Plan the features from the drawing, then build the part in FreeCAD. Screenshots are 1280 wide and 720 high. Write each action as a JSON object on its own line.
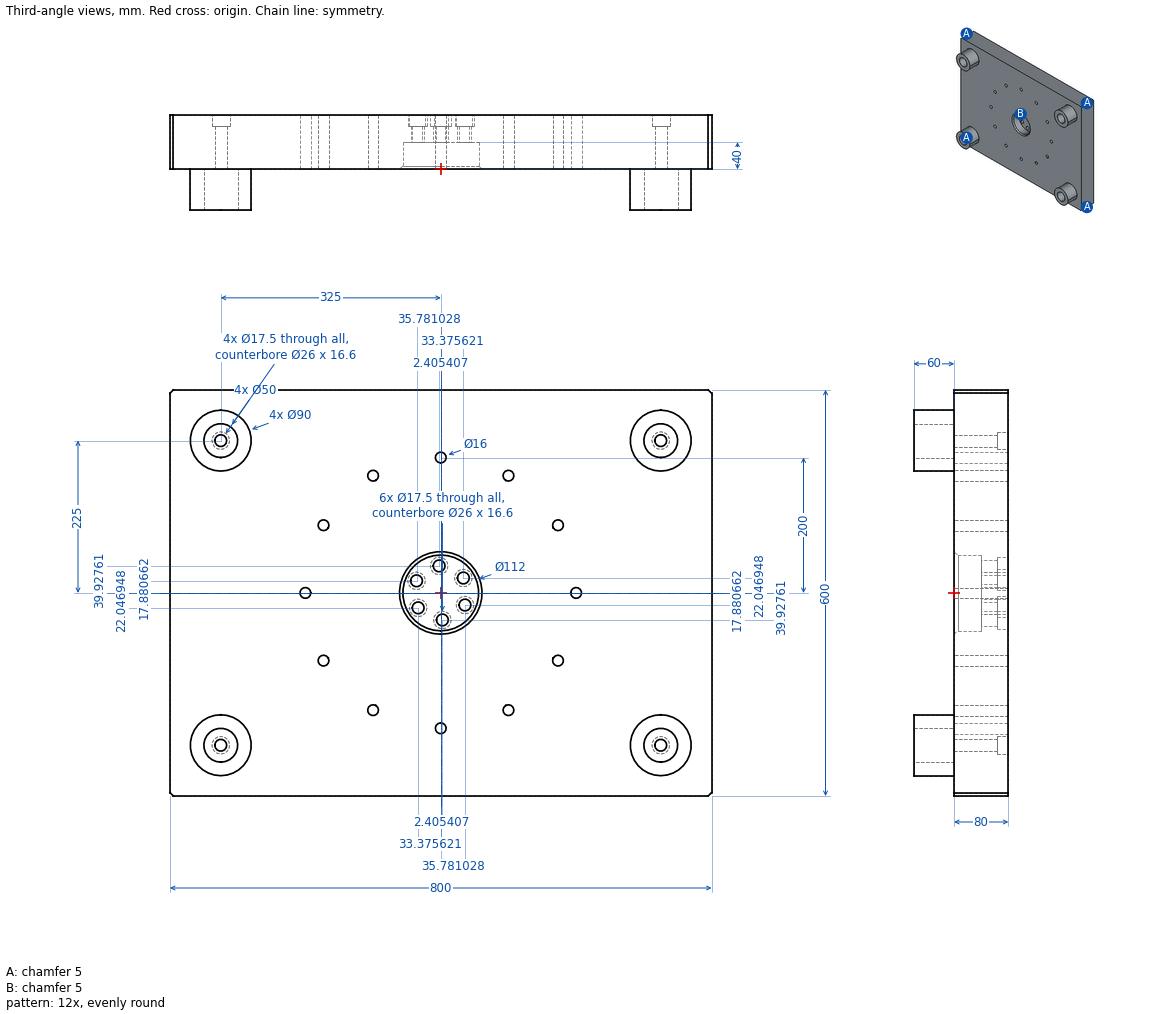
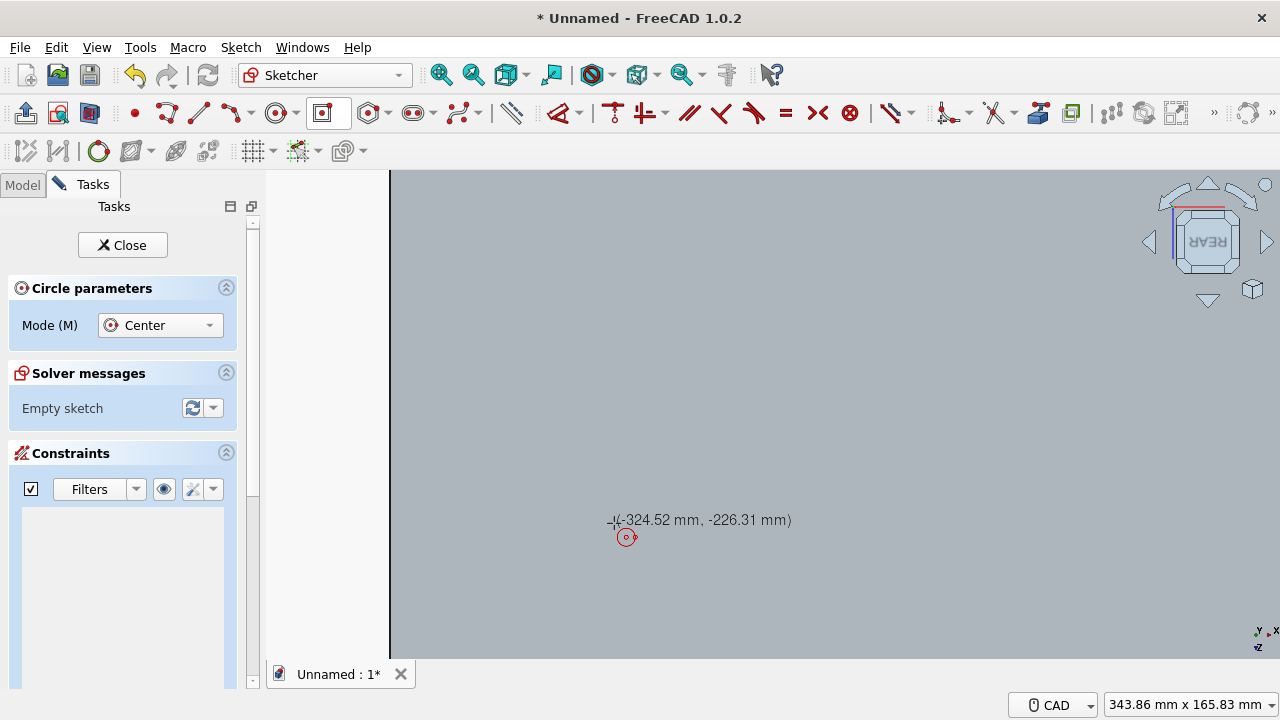
{"action": "scroll", "coordinate": [486, 555], "scroll_direction": "down", "scroll_amount": 8}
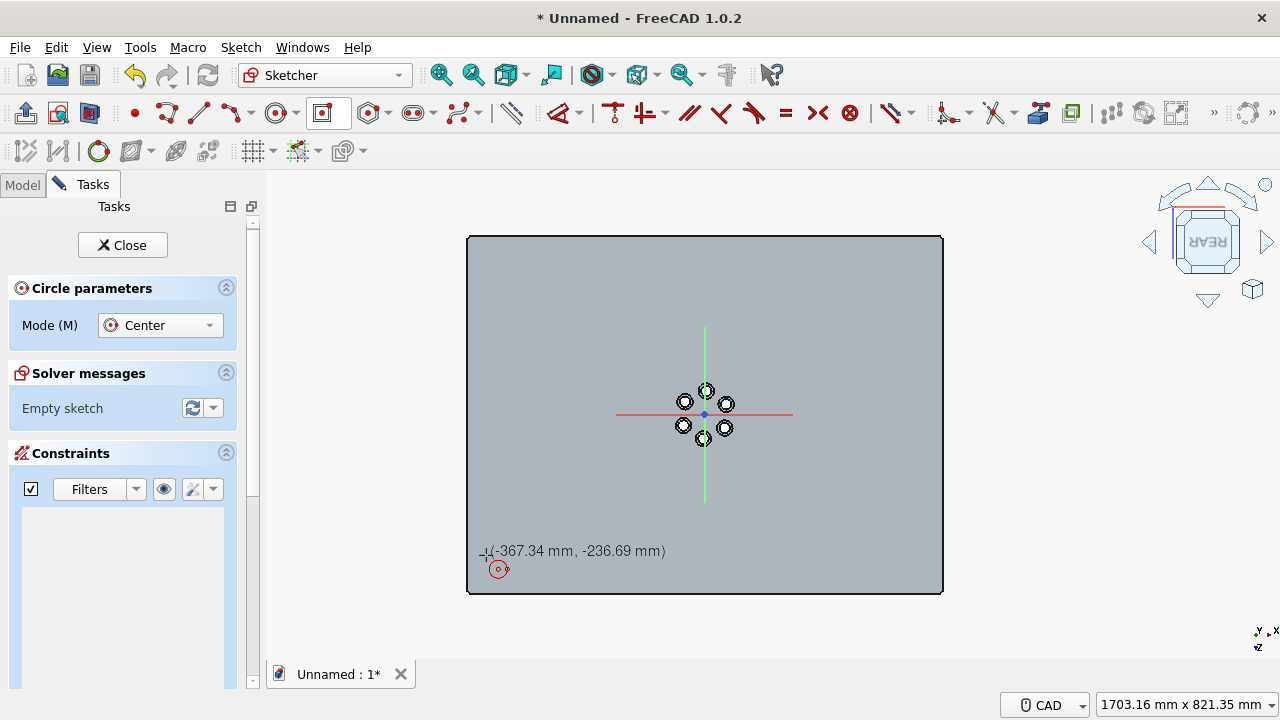
{"action": "left_click", "coordinate": [511, 549]}
{"action": "mouse_move", "coordinate": [515, 545]}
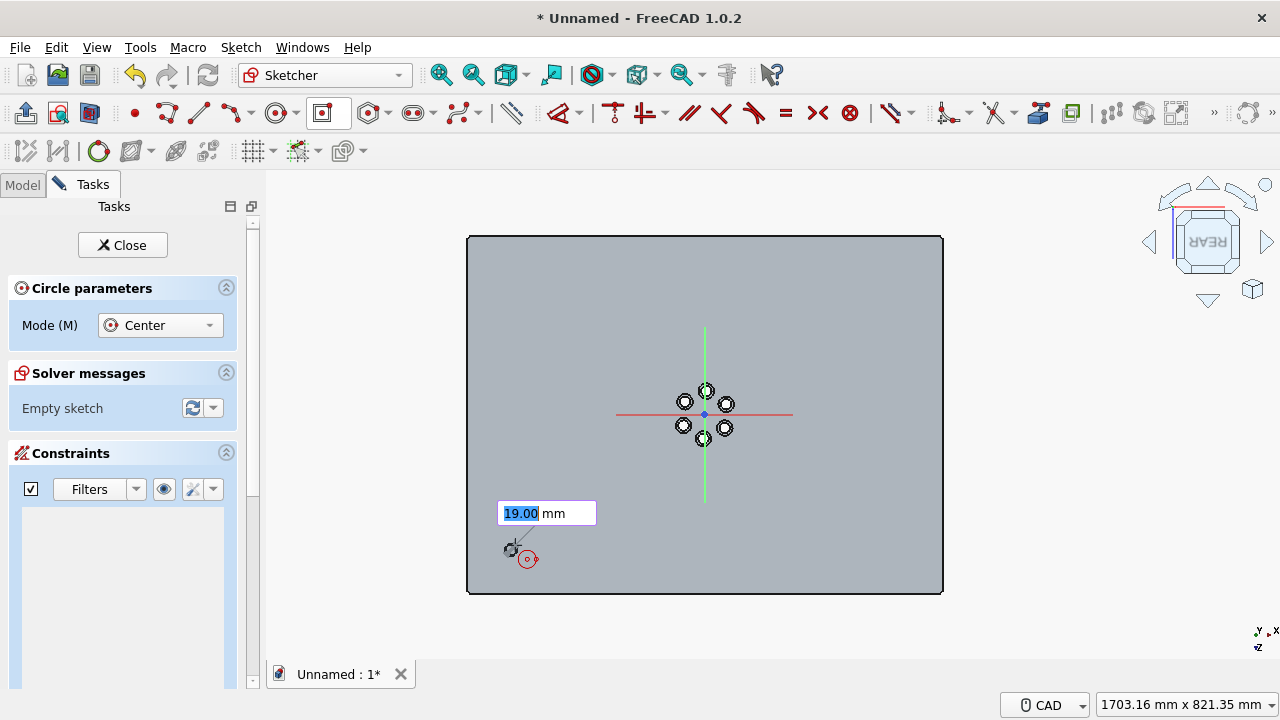
{"action": "type", "text": "17.5"}
{"action": "key", "text": "Return"}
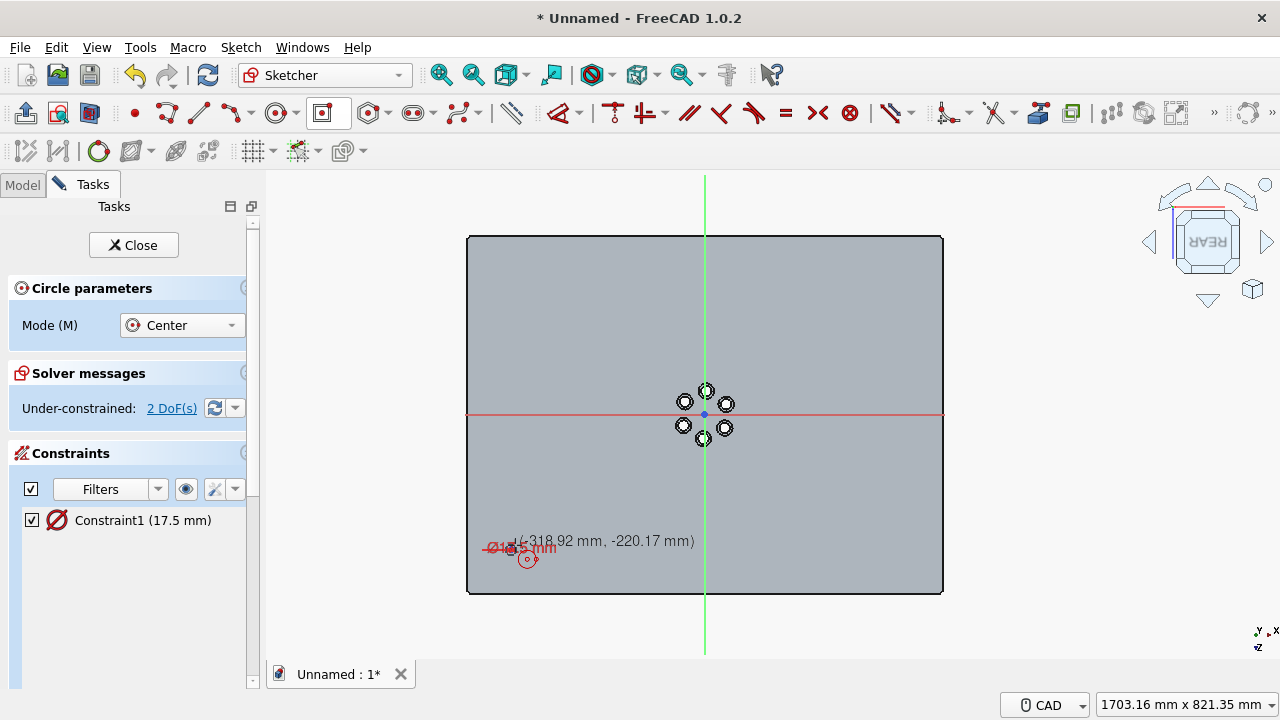
{"action": "scroll", "coordinate": [511, 281], "scroll_direction": "up", "scroll_amount": 8}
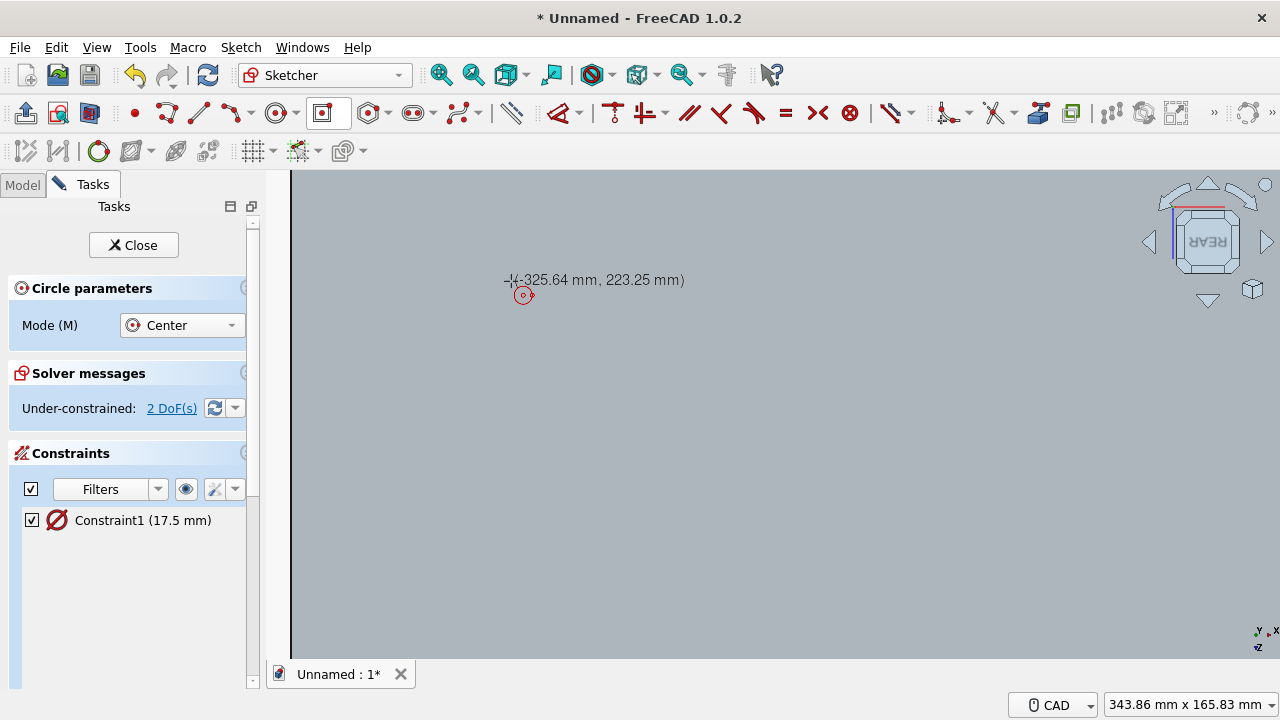
{"action": "scroll", "coordinate": [511, 281], "scroll_direction": "down", "scroll_amount": 8}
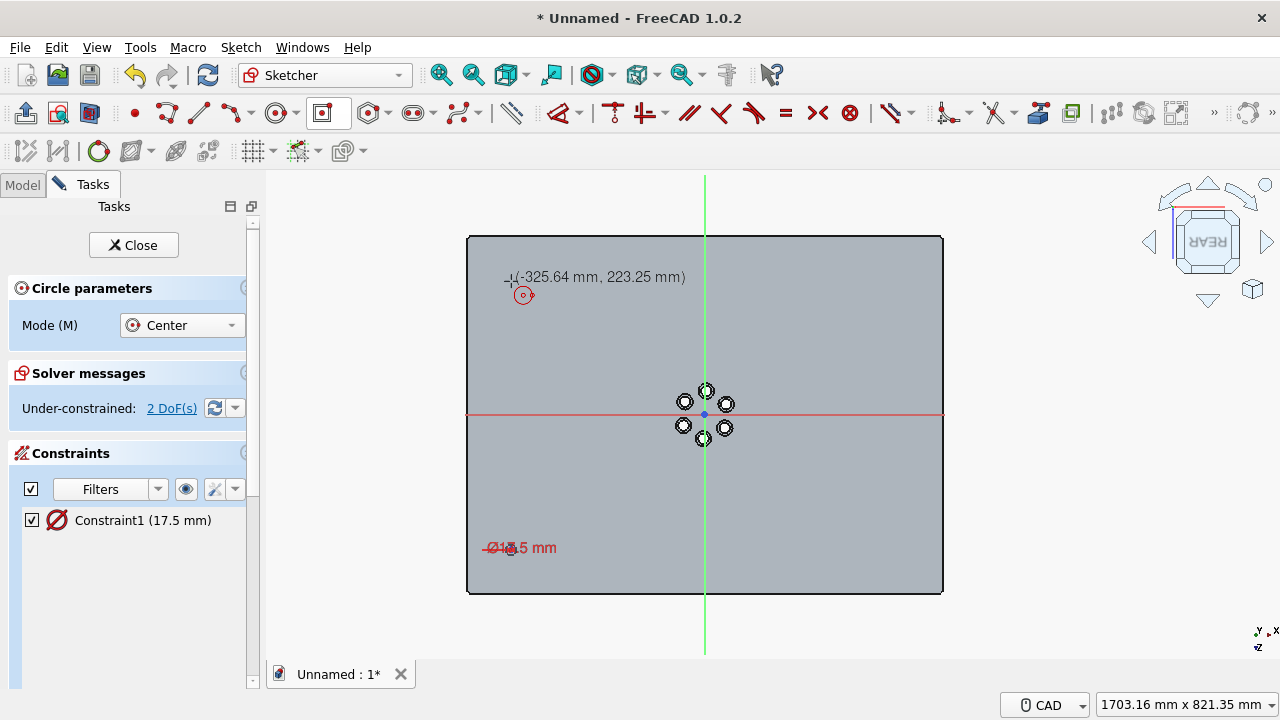
{"action": "left_click", "coordinate": [511, 281]}
{"action": "mouse_move", "coordinate": [515, 277]}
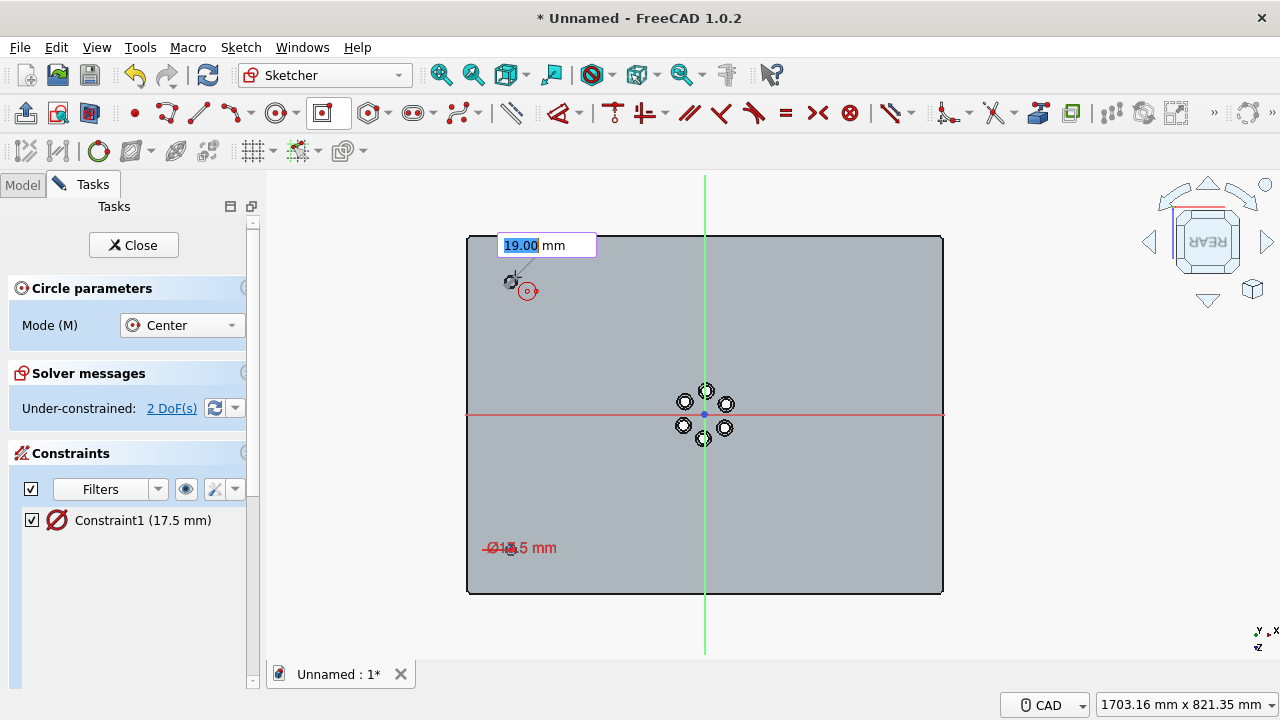
{"action": "type", "text": "17.5"}
{"action": "key", "text": "Return"}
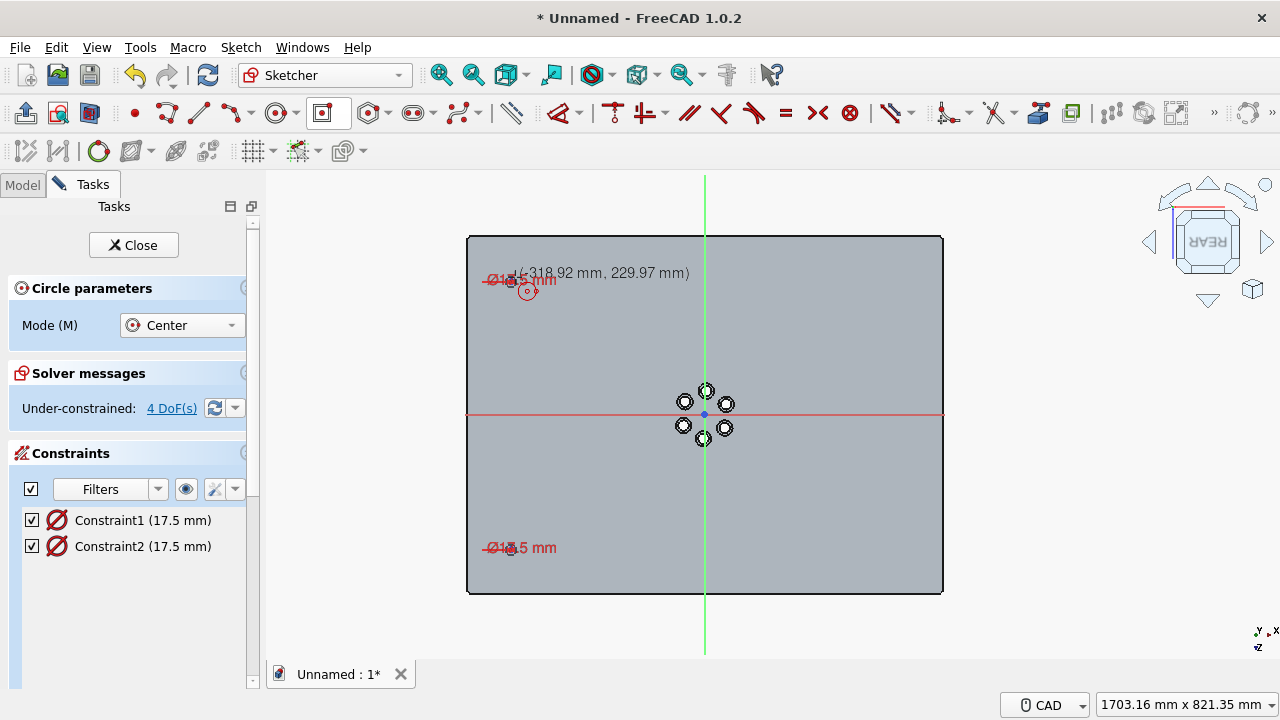
{"action": "scroll", "coordinate": [898, 281], "scroll_direction": "up", "scroll_amount": 8}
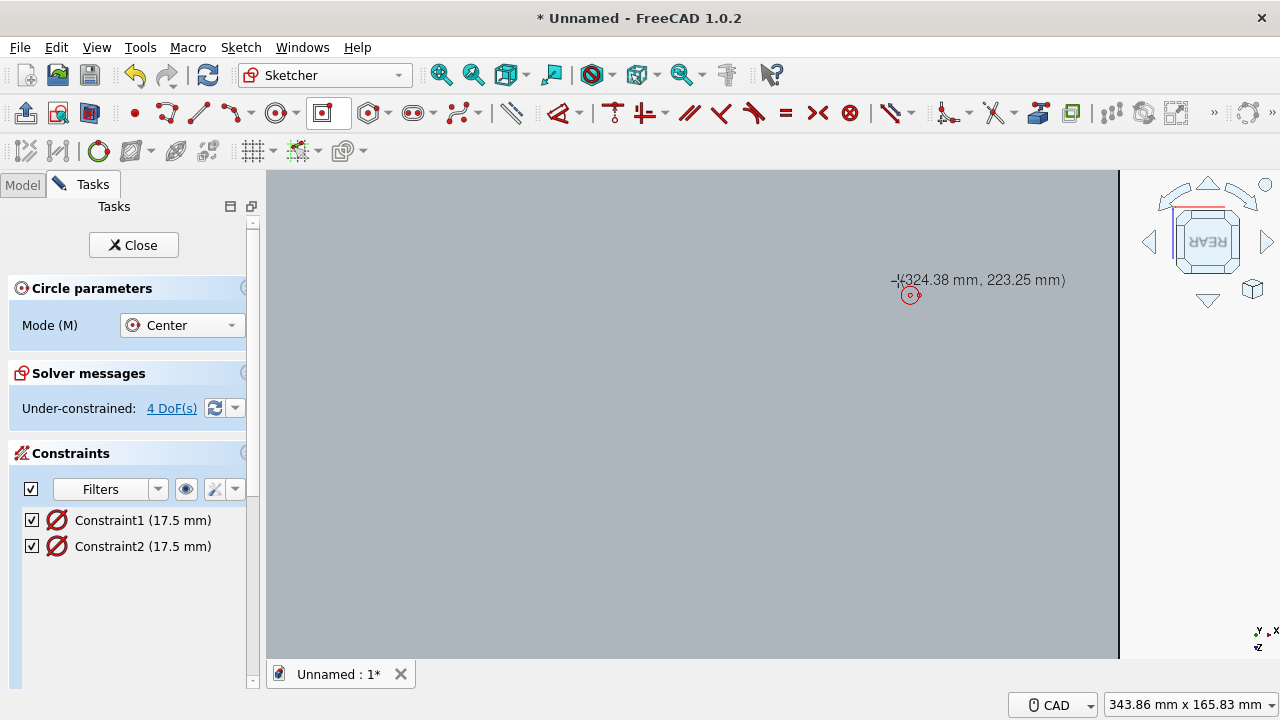
{"action": "scroll", "coordinate": [898, 281], "scroll_direction": "down", "scroll_amount": 8}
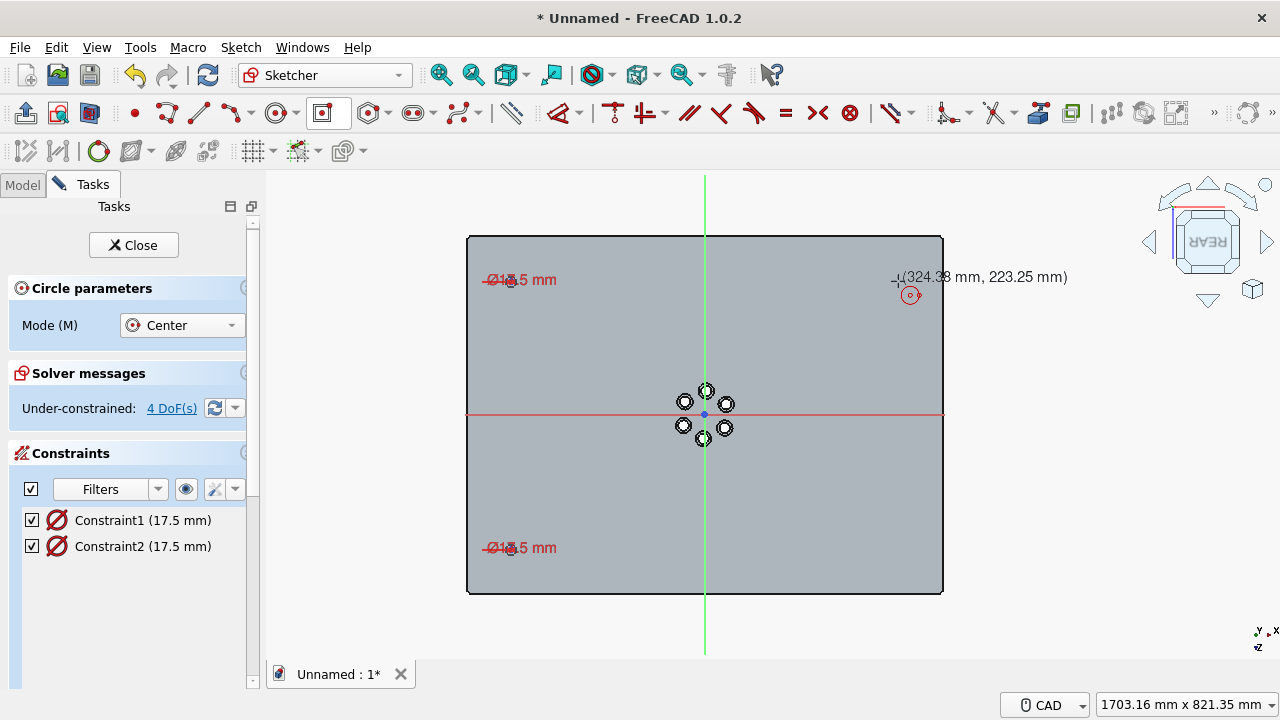
{"action": "left_click", "coordinate": [898, 281]}
{"action": "mouse_move", "coordinate": [902, 277]}